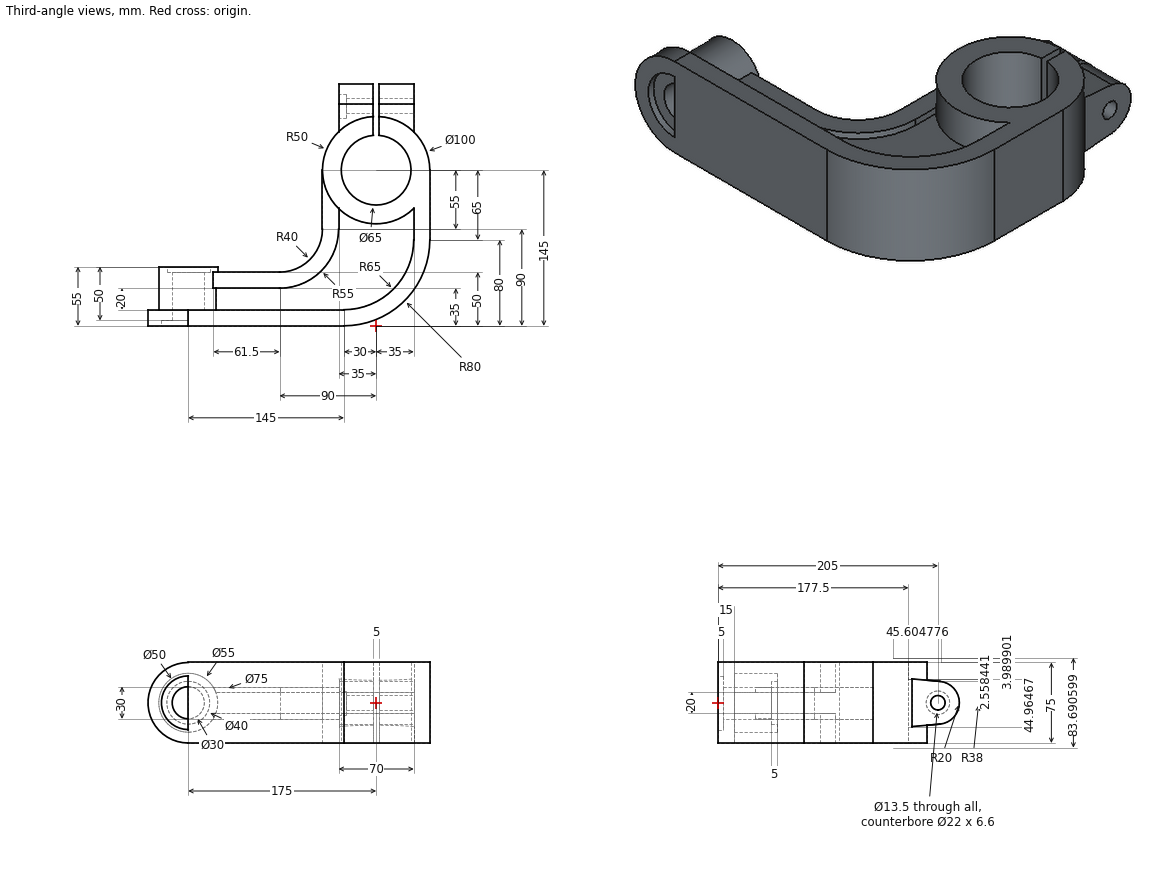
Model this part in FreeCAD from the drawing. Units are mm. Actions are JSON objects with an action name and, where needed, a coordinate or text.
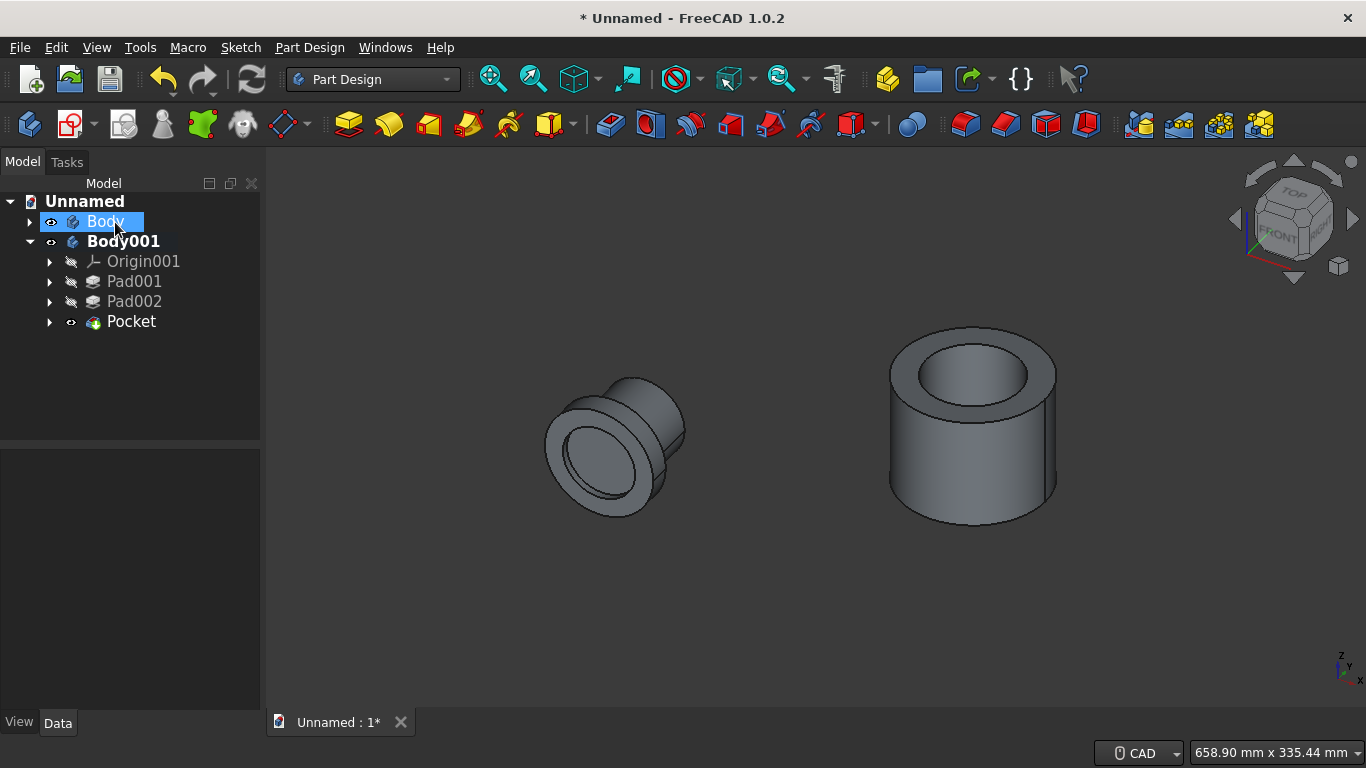
{"action": "key", "text": "v f"}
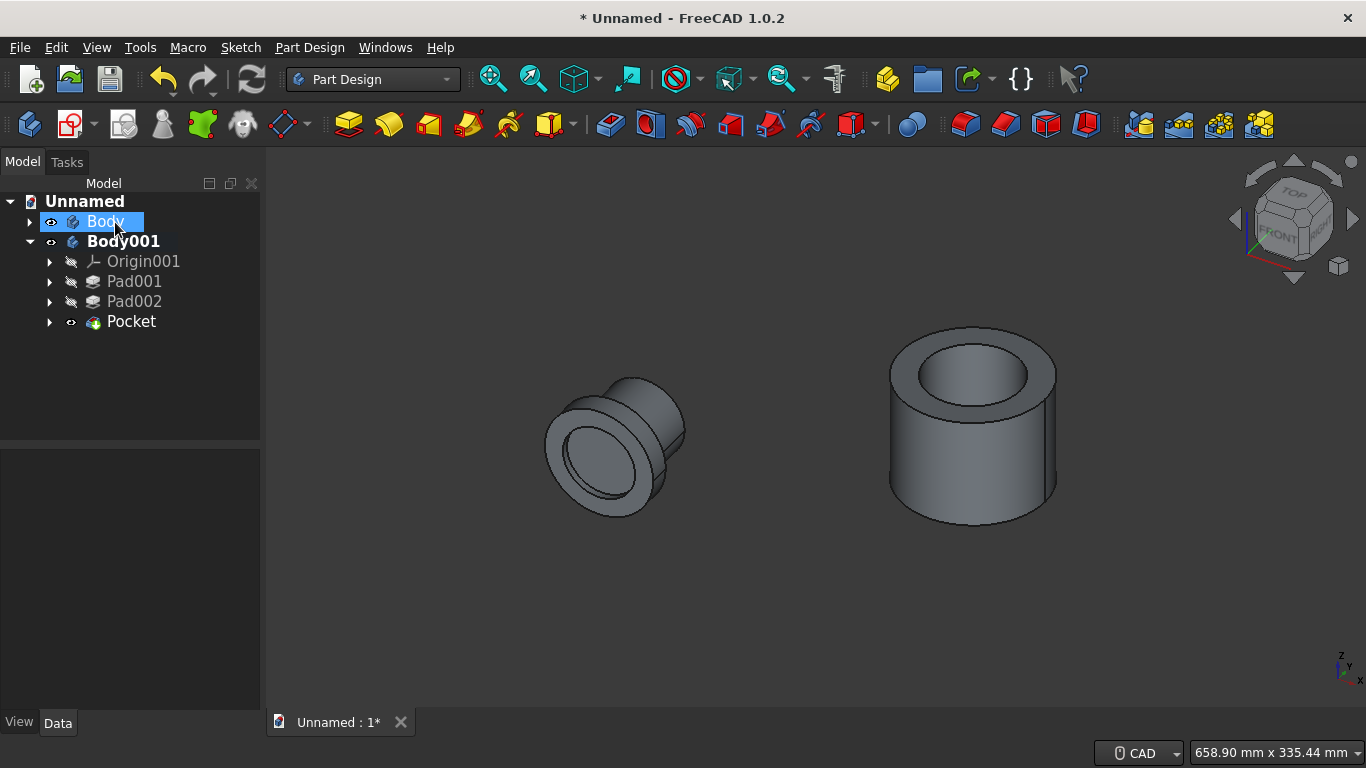
{"action": "key", "text": "4"}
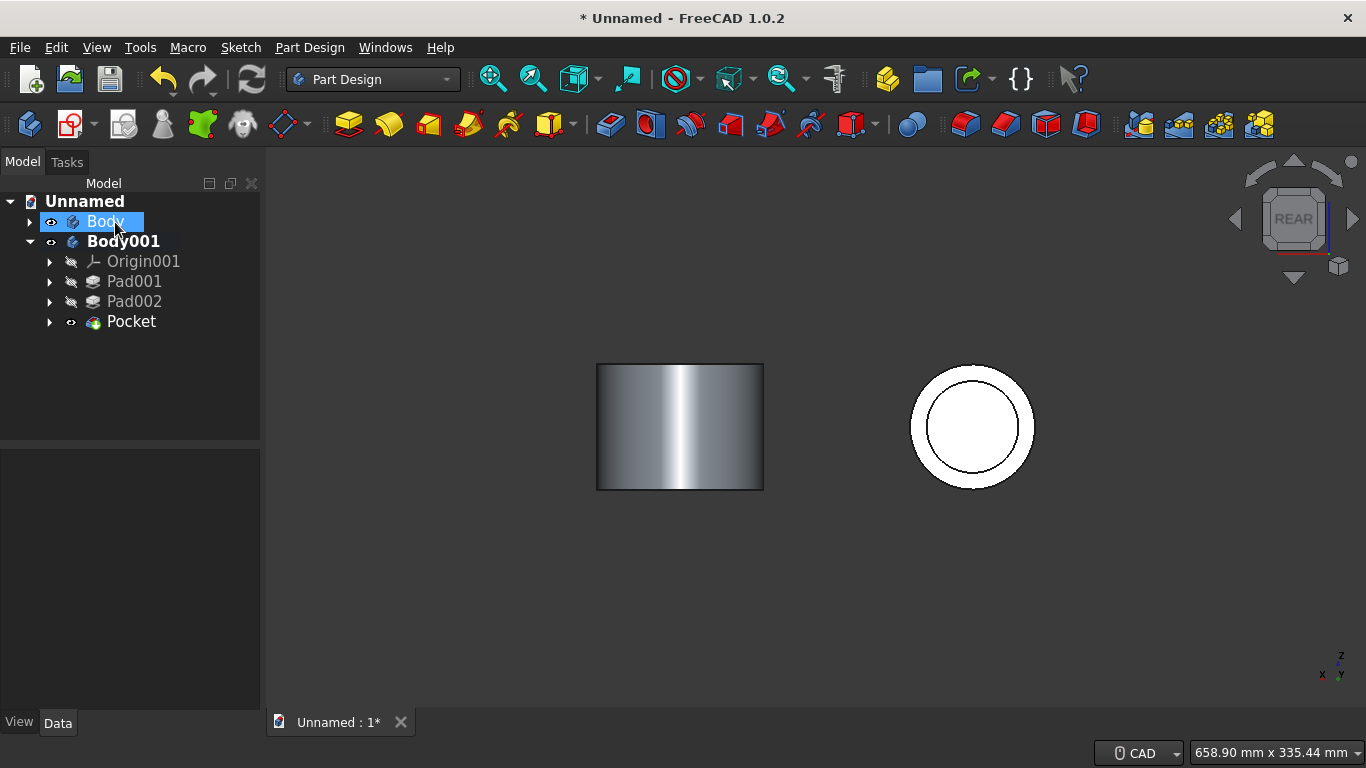
{"action": "key", "text": "v f"}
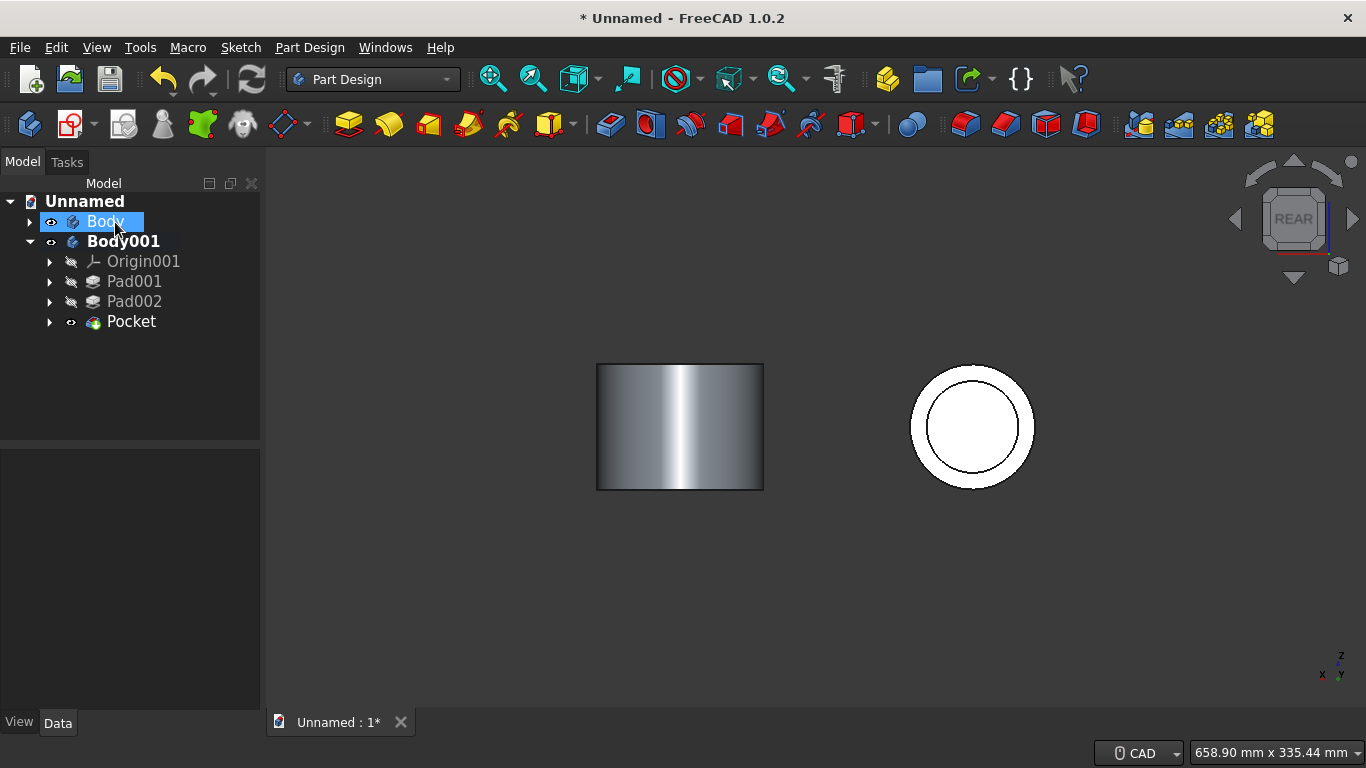
{"action": "left_click", "coordinate": [973, 426]}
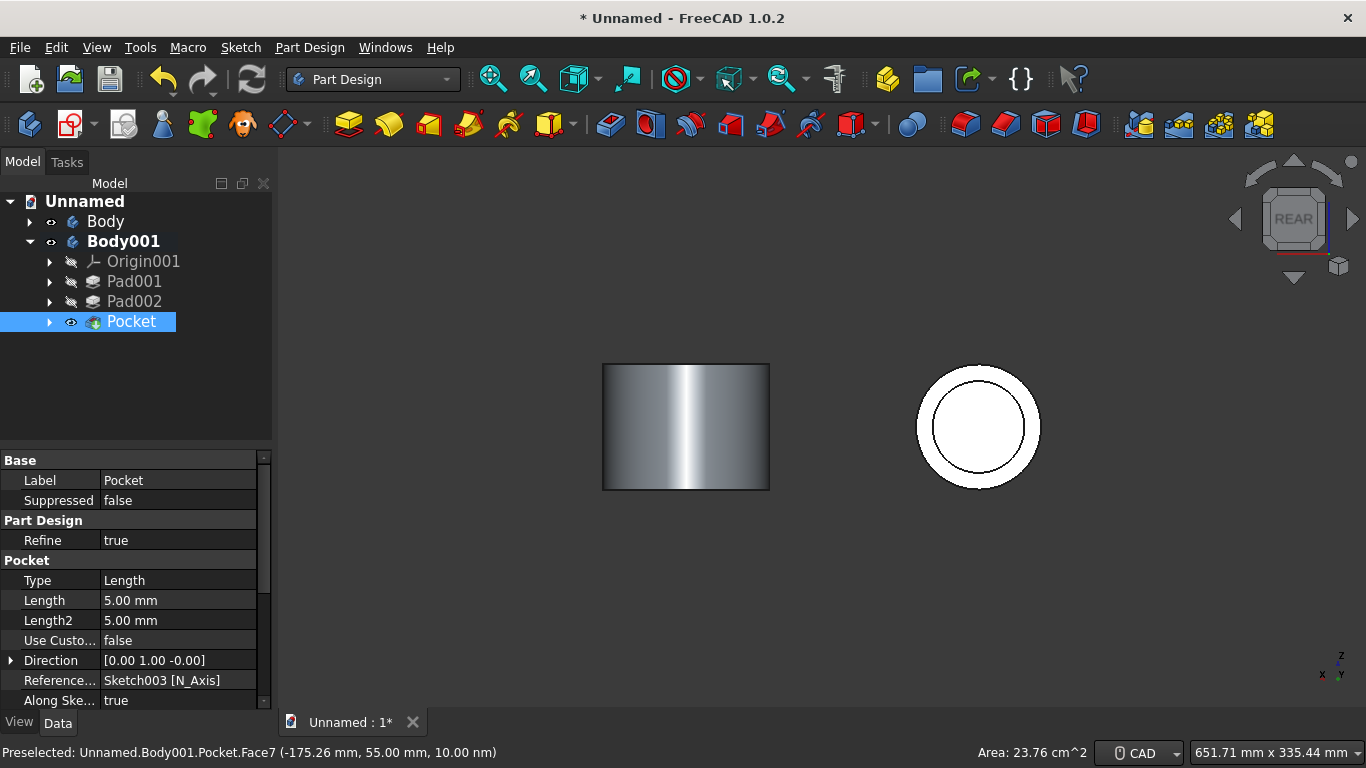
{"action": "left_click", "coordinate": [70, 124]}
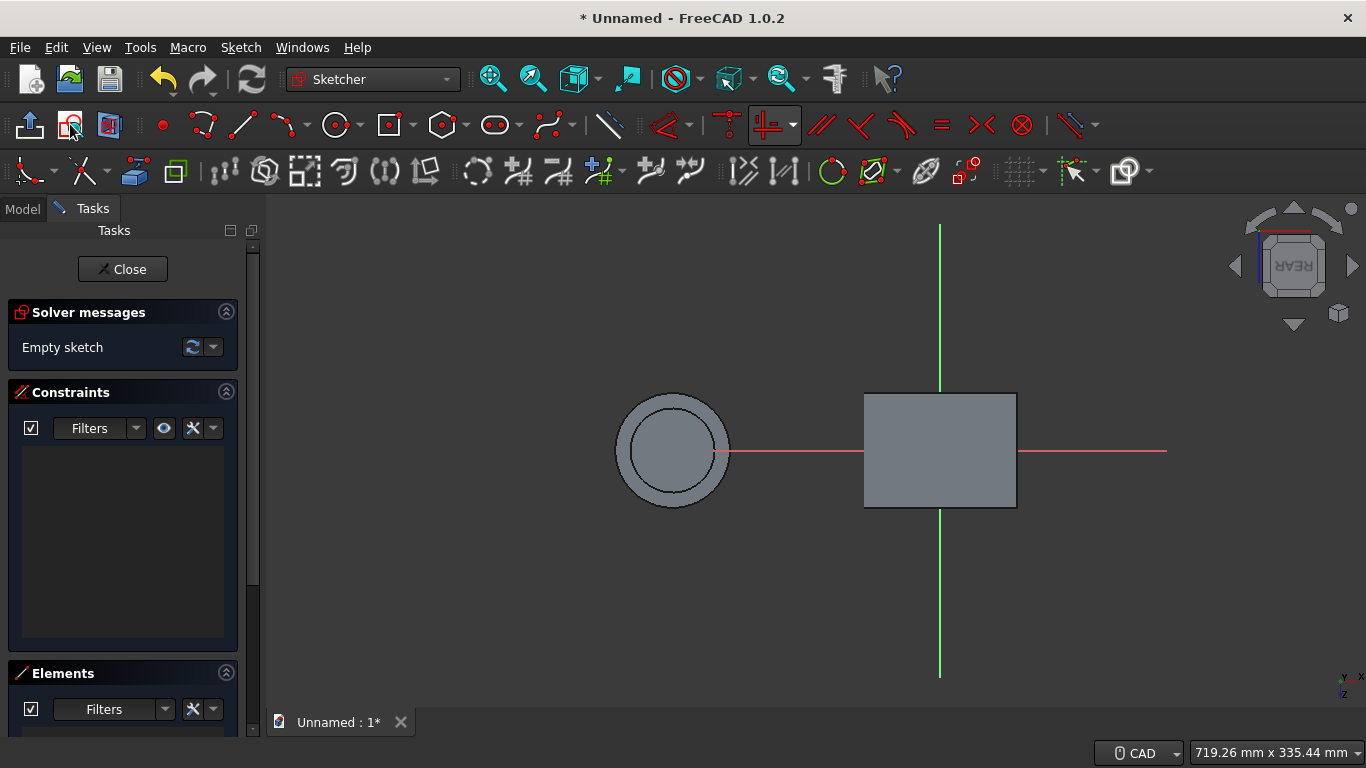
{"action": "scroll", "coordinate": [661, 450], "scroll_direction": "up", "scroll_amount": 10}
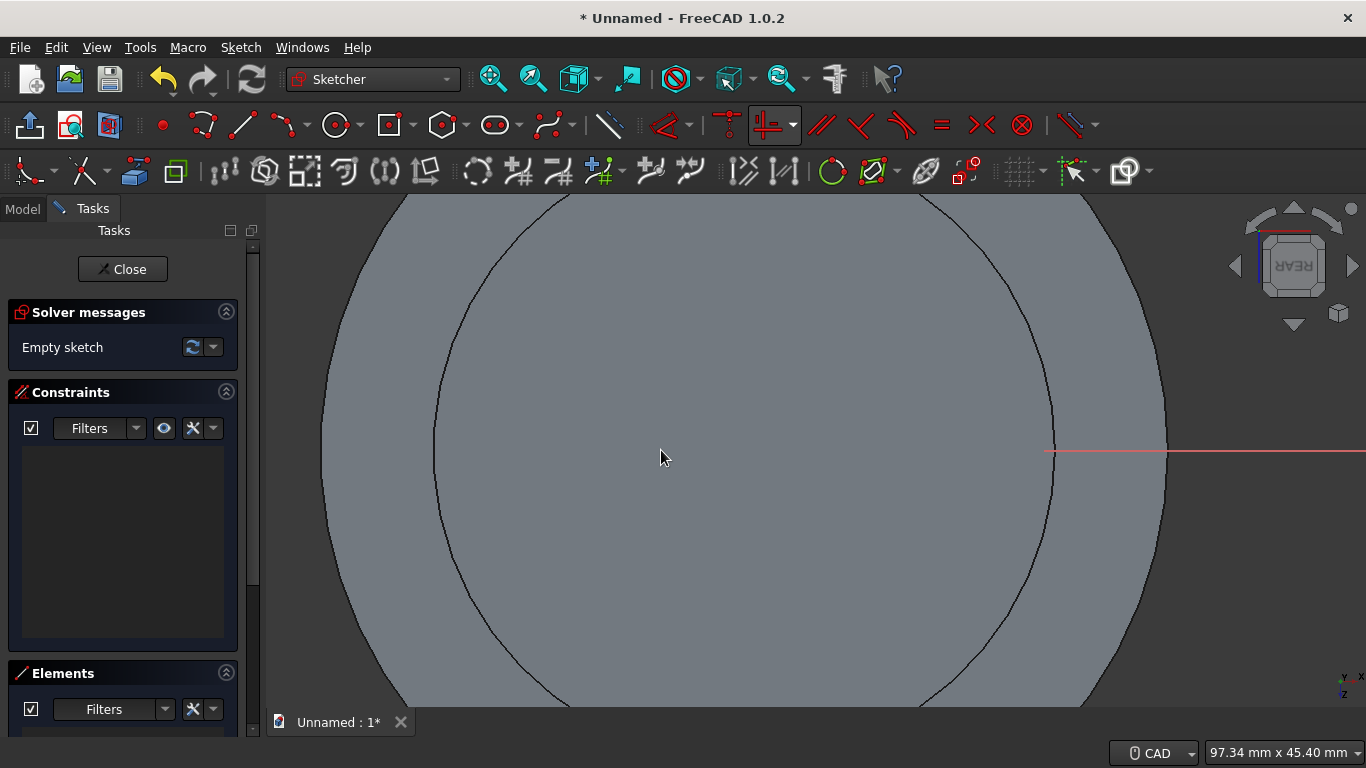
{"action": "left_click", "coordinate": [336, 126]}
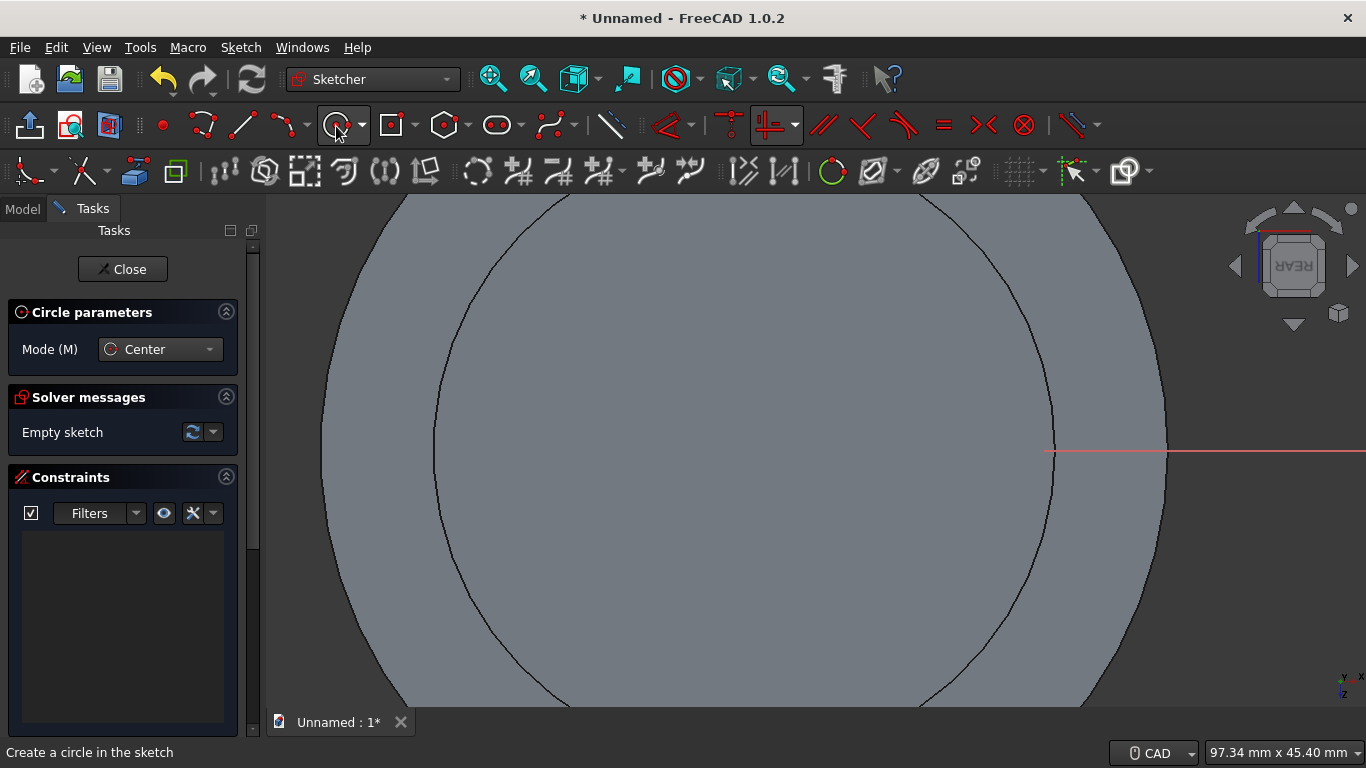
{"action": "left_click", "coordinate": [744, 450]}
{"action": "left_click", "coordinate": [864, 331]}
{"action": "key", "text": "Escape"}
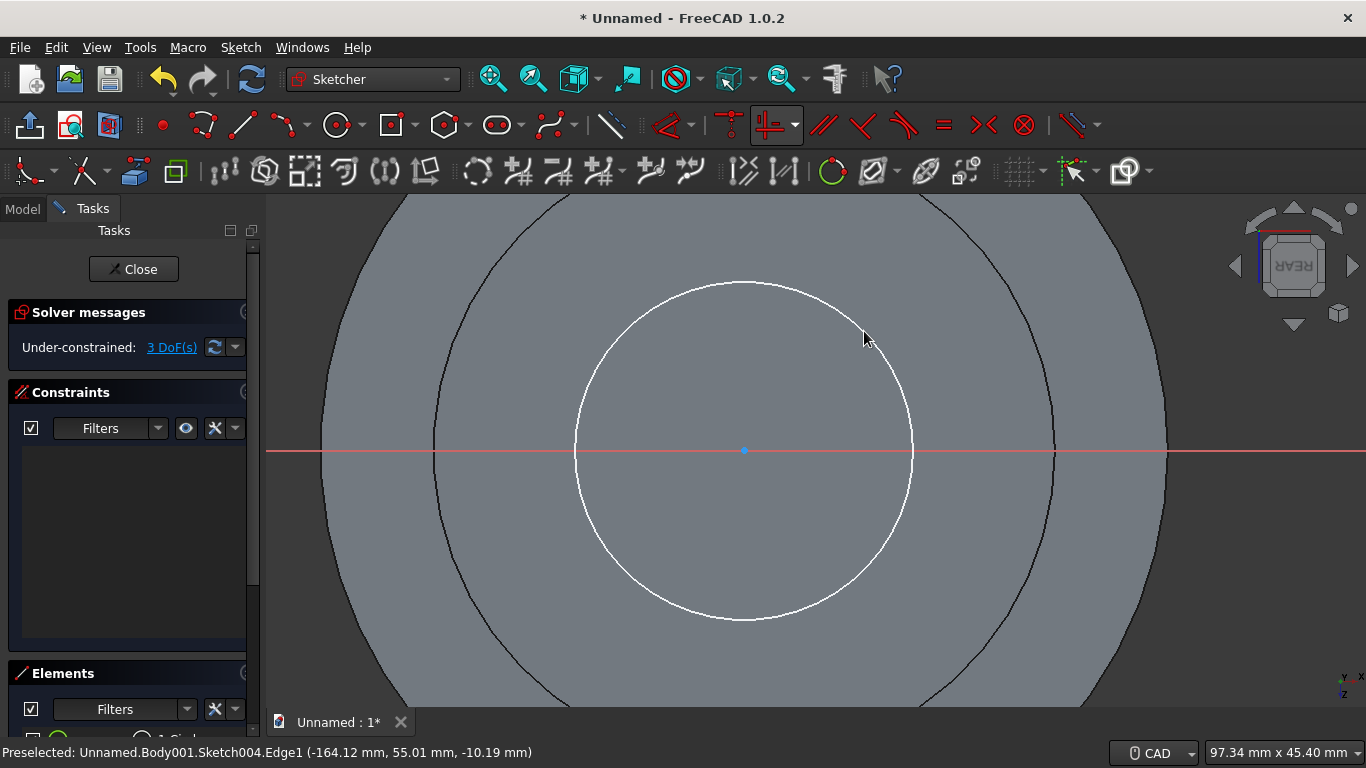
{"action": "left_click", "coordinate": [744, 451]}